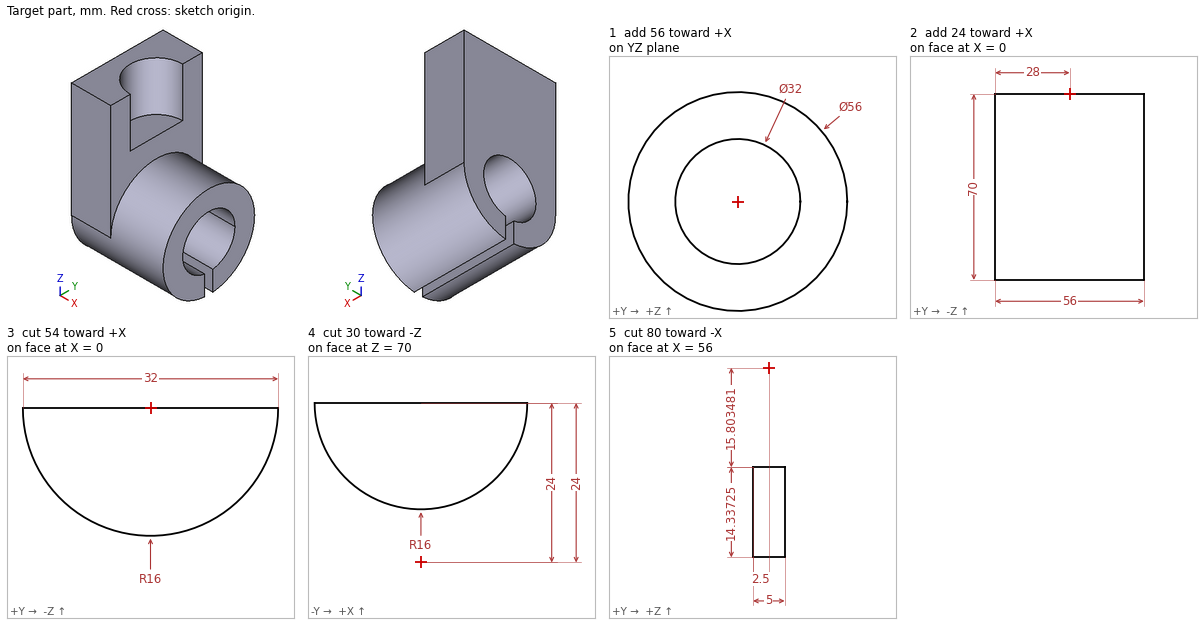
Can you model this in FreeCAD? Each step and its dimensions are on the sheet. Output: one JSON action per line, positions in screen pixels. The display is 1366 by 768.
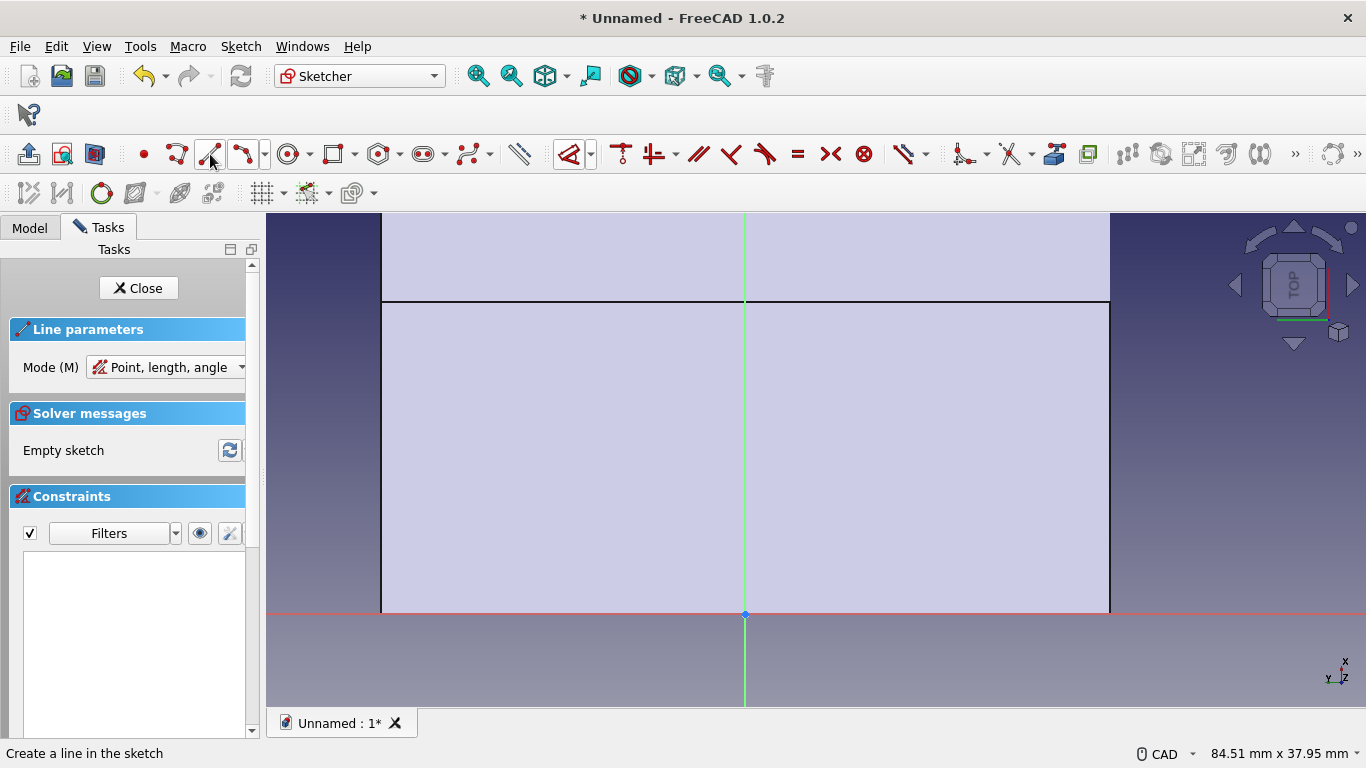
{"action": "left_click", "coordinate": [953, 302]}
{"action": "left_click", "coordinate": [537, 302]}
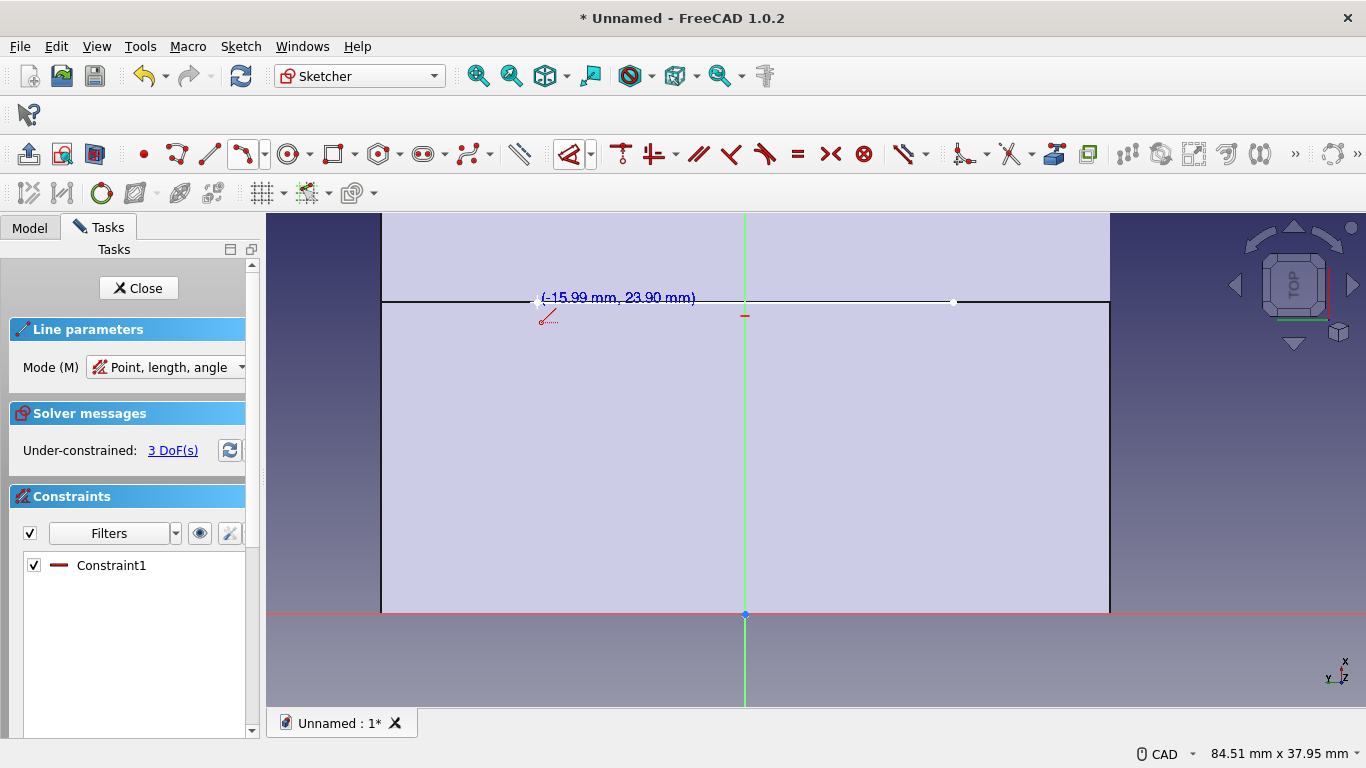
{"action": "left_click", "coordinate": [242, 154]}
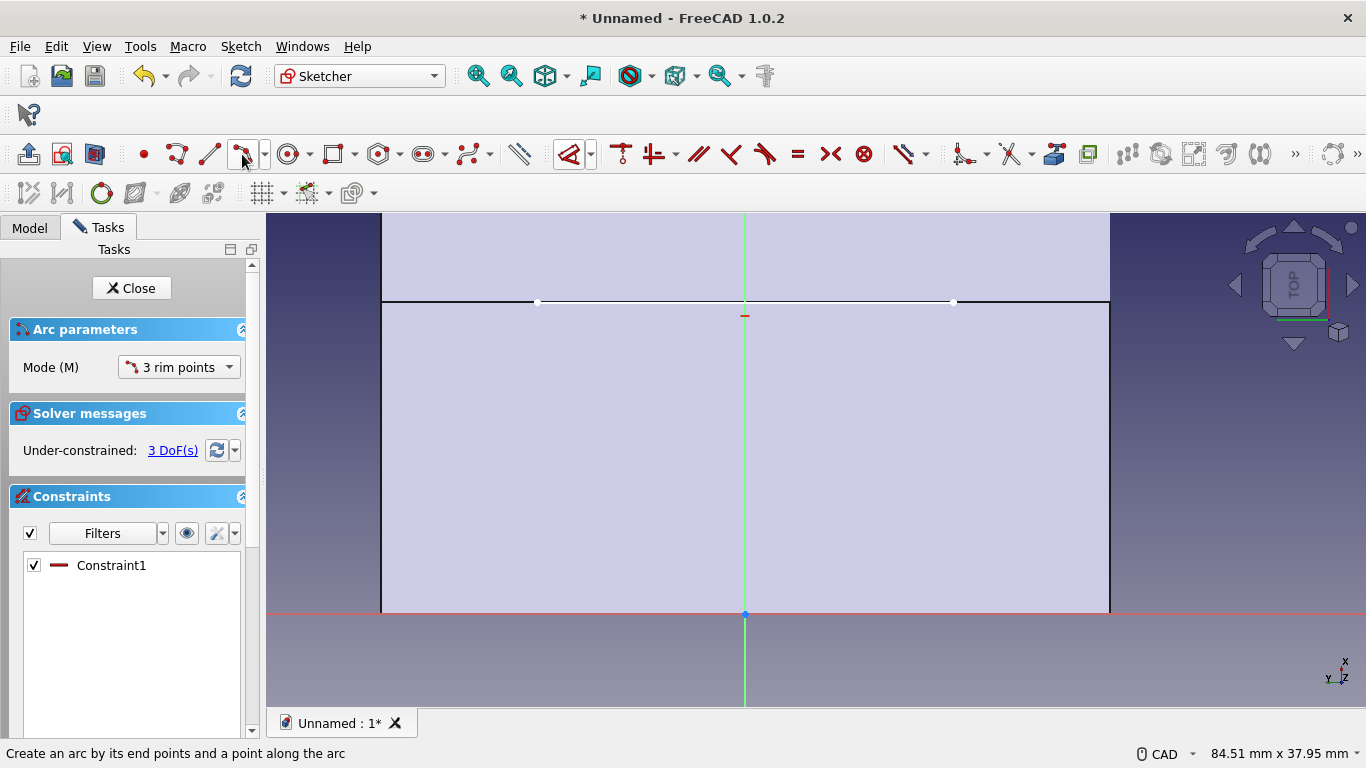
{"action": "left_click", "coordinate": [537, 303]}
{"action": "left_click", "coordinate": [953, 303]}
{"action": "left_click", "coordinate": [681, 500]}
{"action": "key", "text": "Escape"}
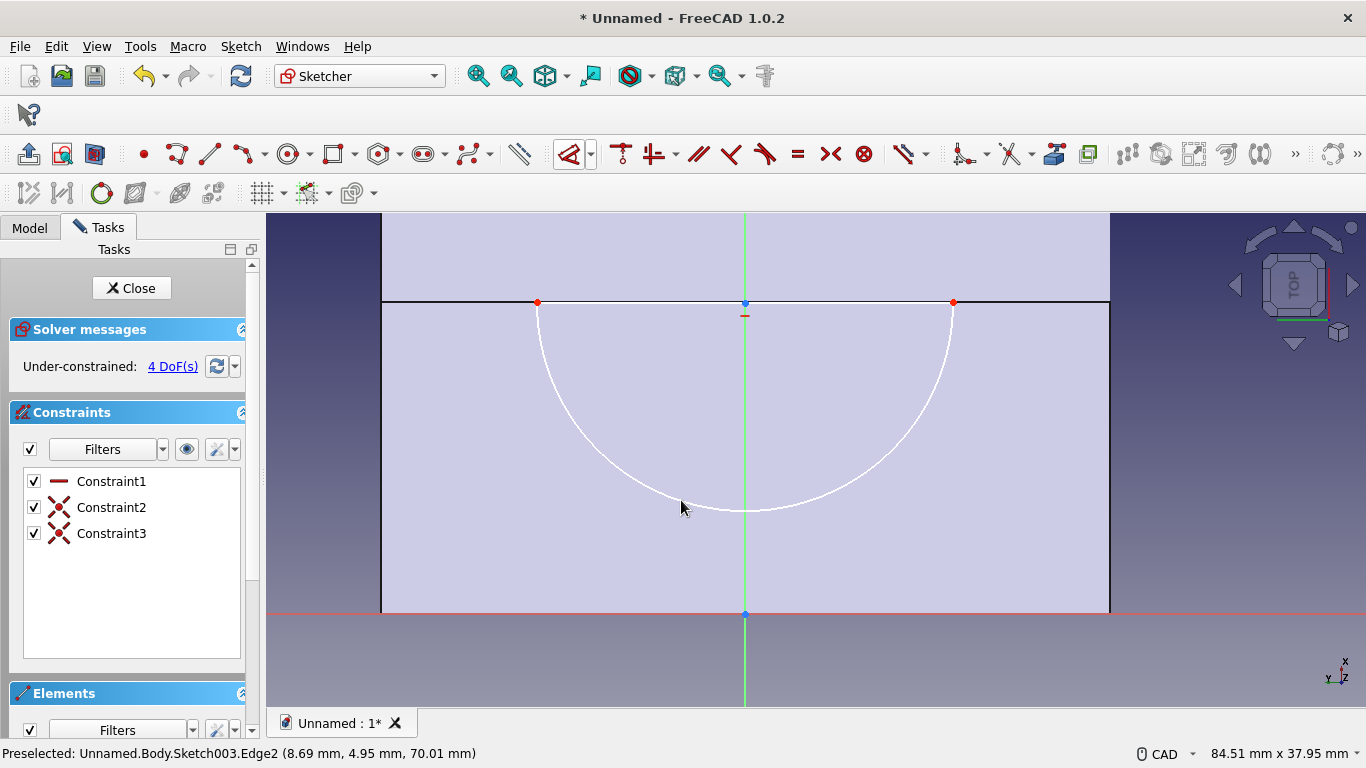
{"action": "left_click", "coordinate": [745, 303]}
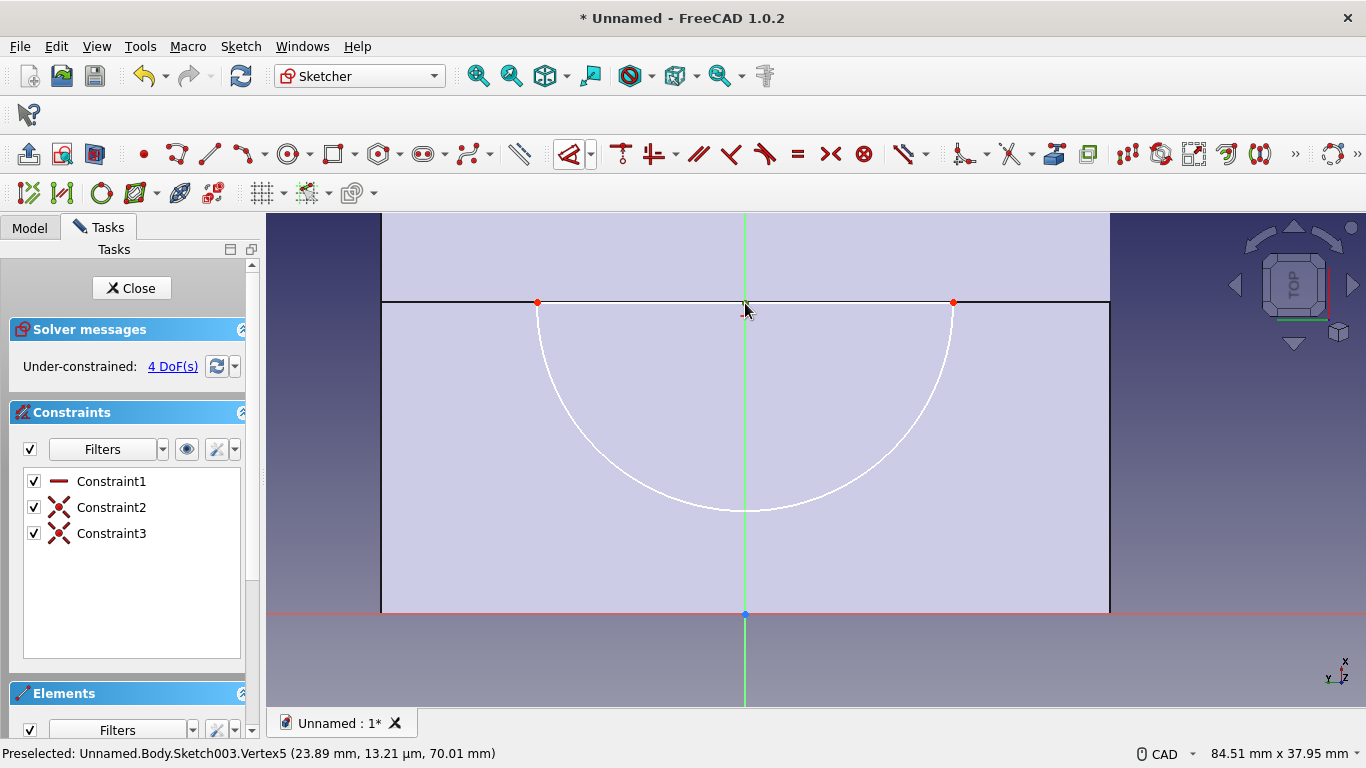
{"action": "left_click", "coordinate": [745, 648]}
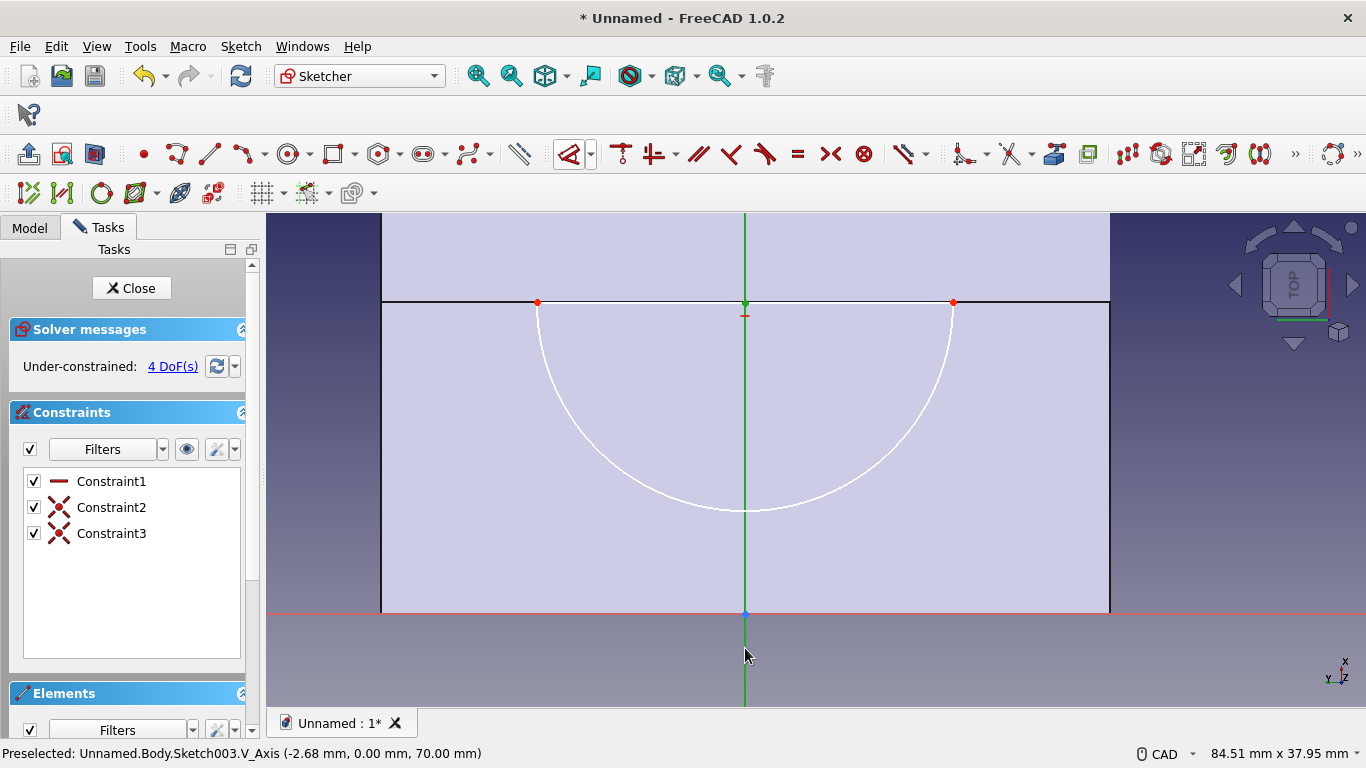
{"action": "key", "text": "c"}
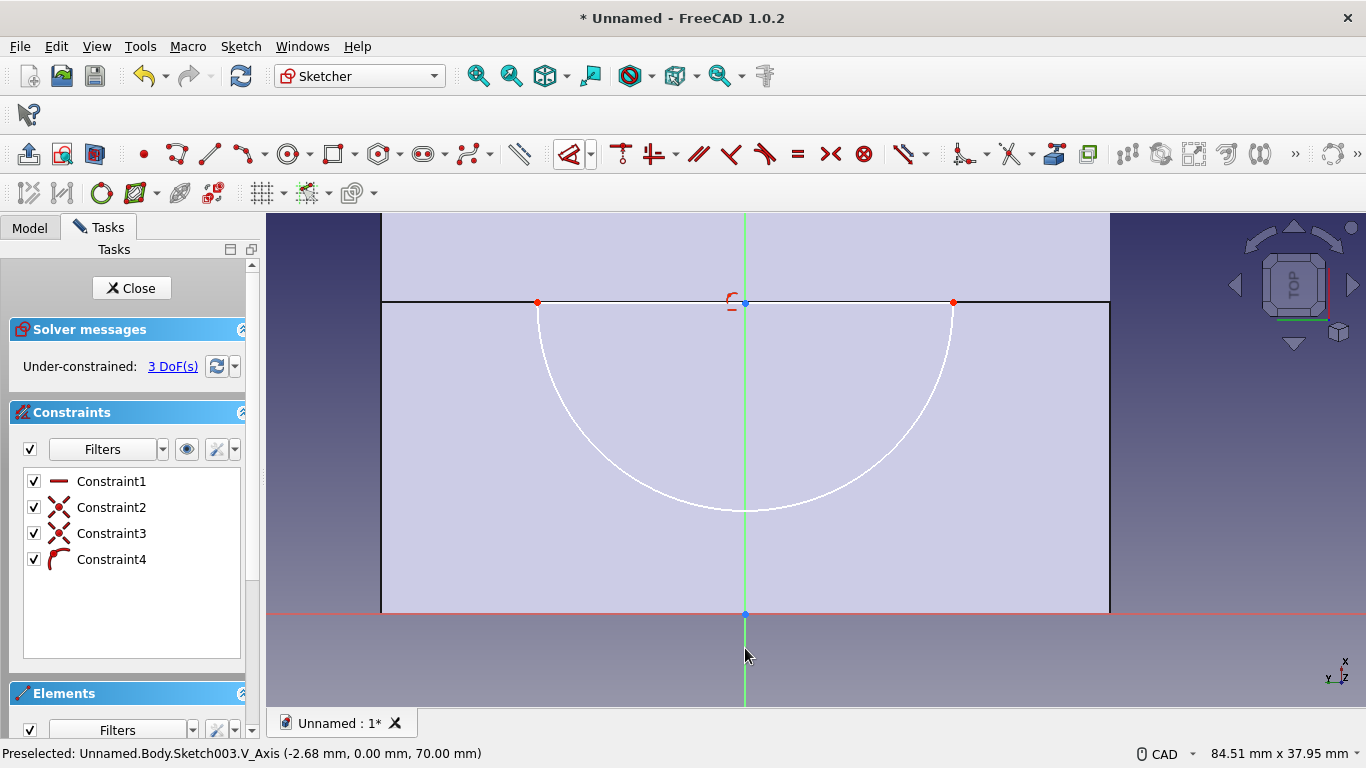
{"action": "left_click", "coordinate": [623, 471]}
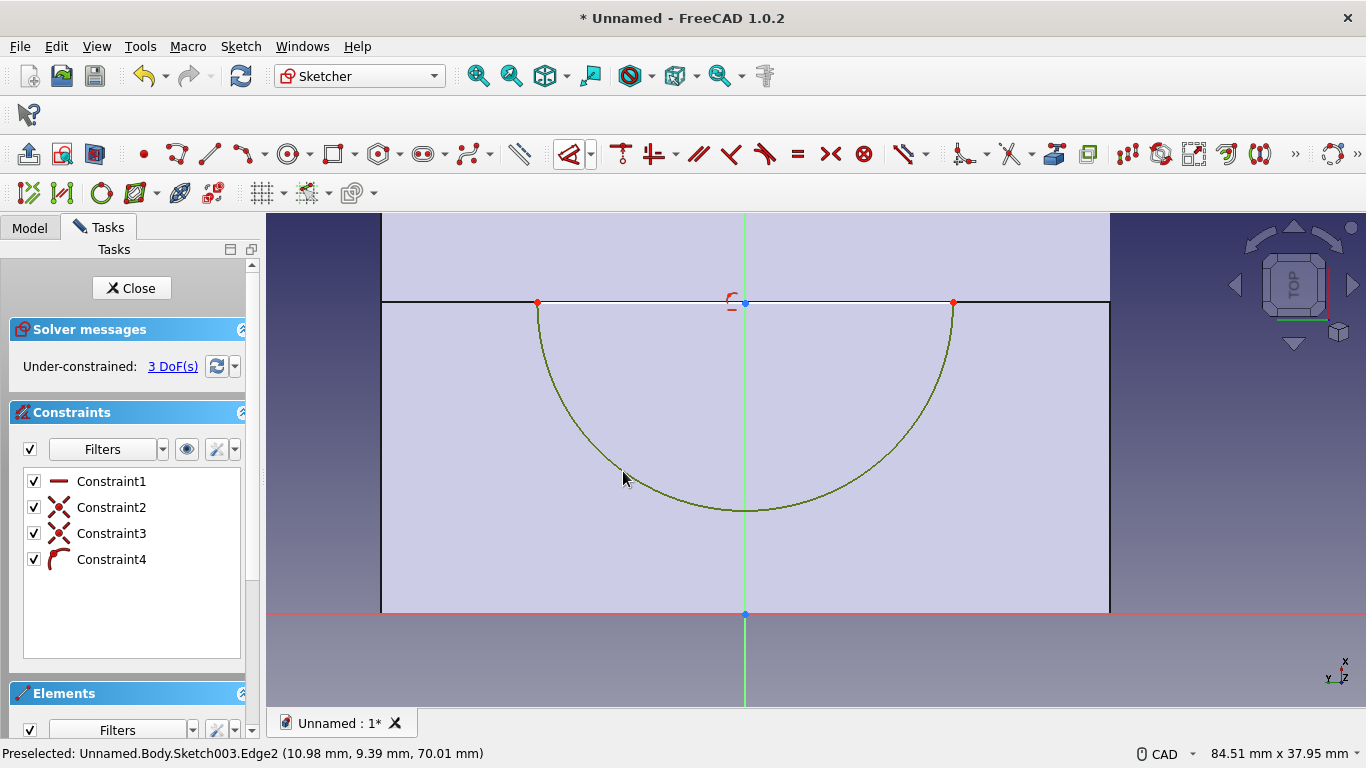
{"action": "key", "text": "k r"}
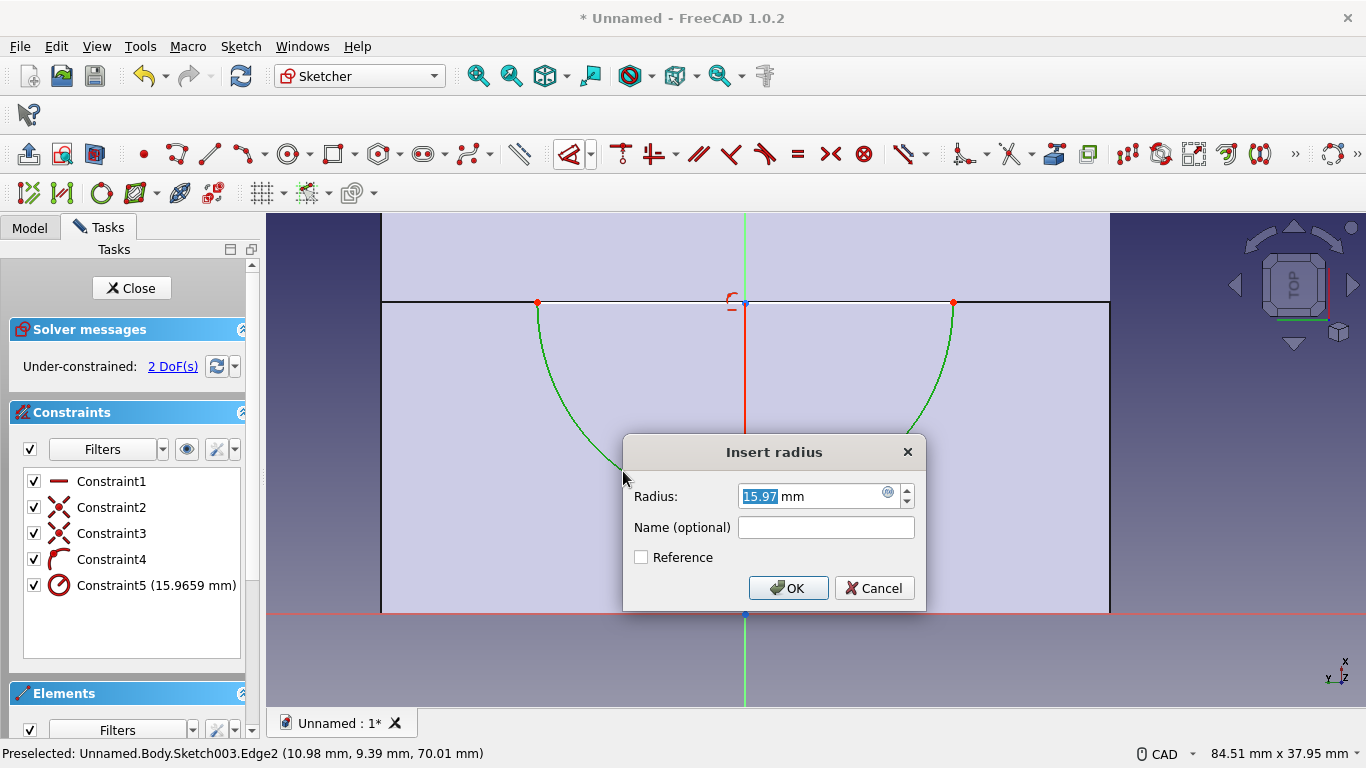
{"action": "type", "text": "16"}
{"action": "key", "text": "Return"}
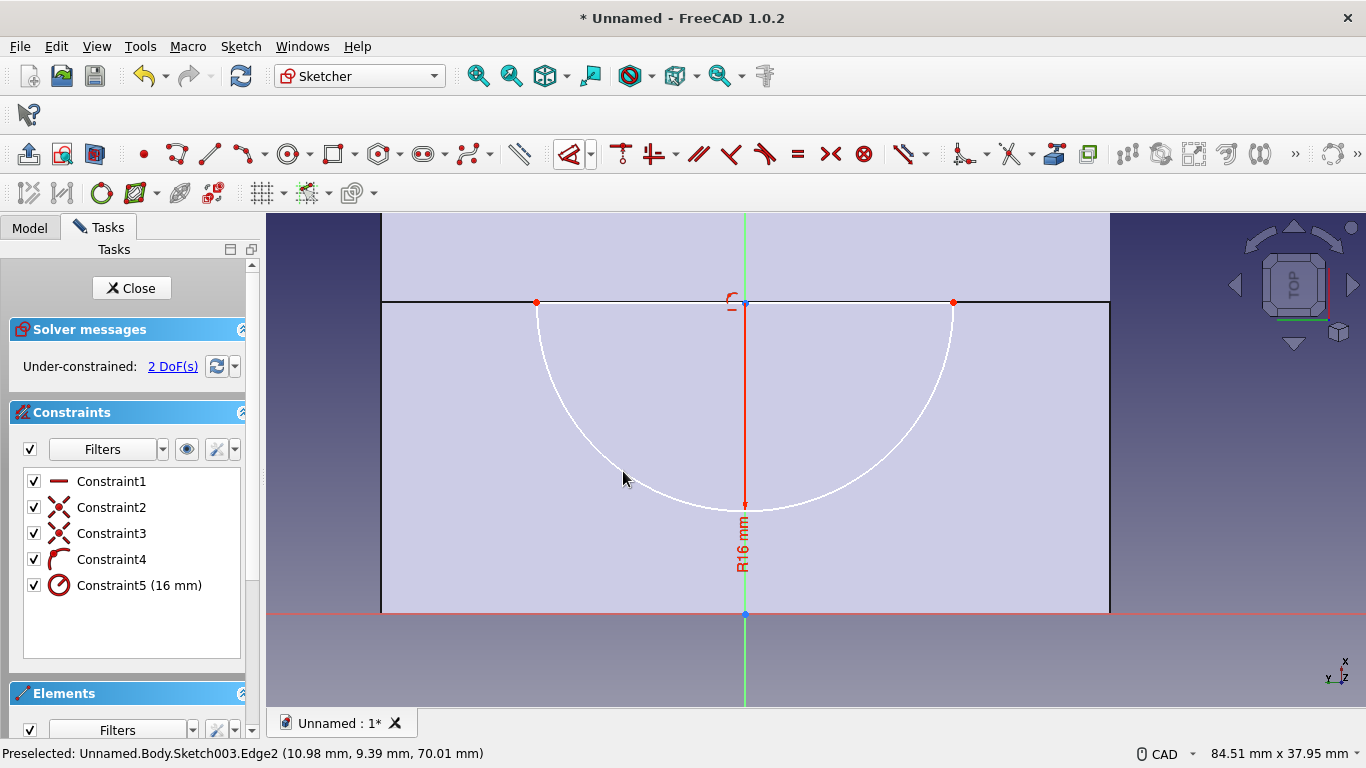
{"action": "left_click", "coordinate": [953, 303]}